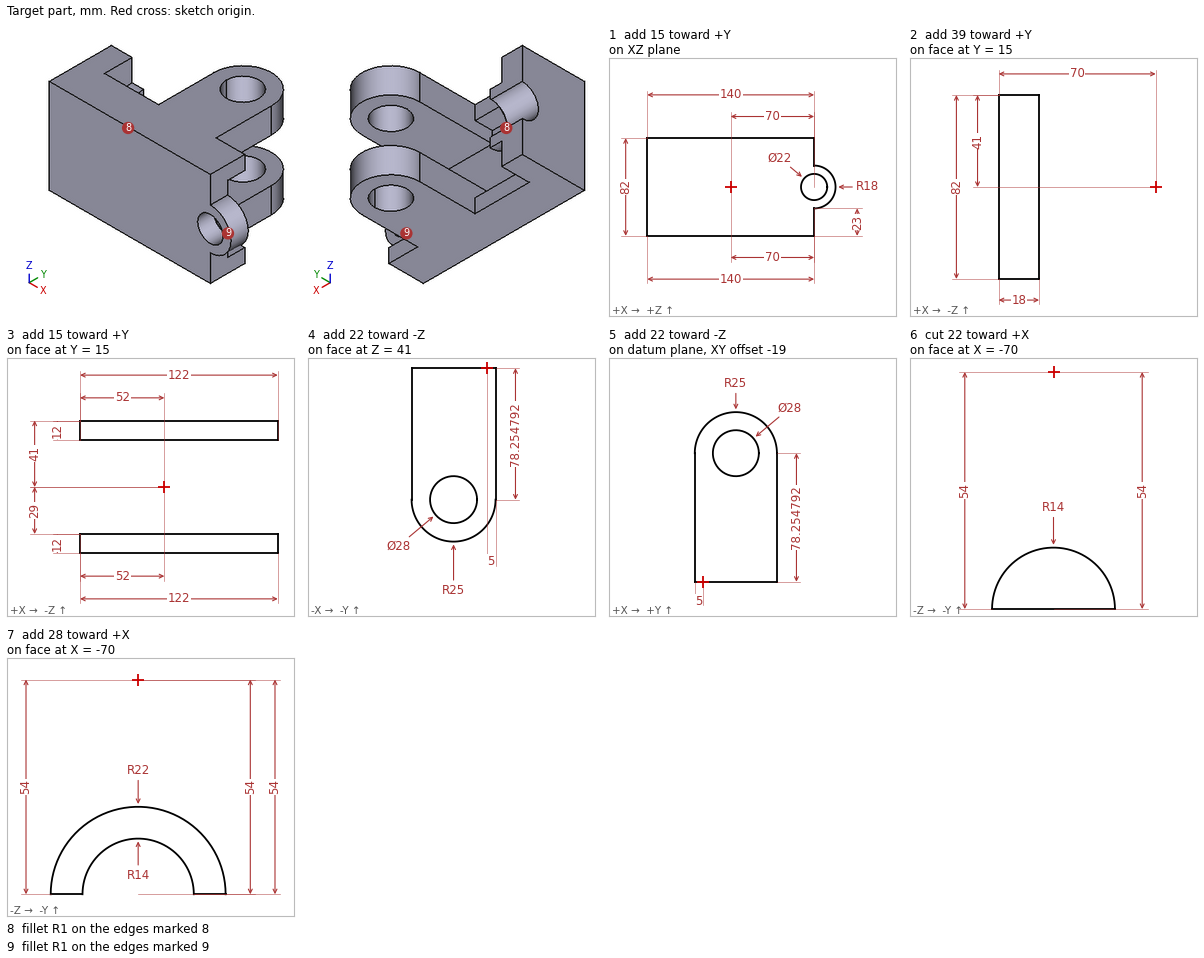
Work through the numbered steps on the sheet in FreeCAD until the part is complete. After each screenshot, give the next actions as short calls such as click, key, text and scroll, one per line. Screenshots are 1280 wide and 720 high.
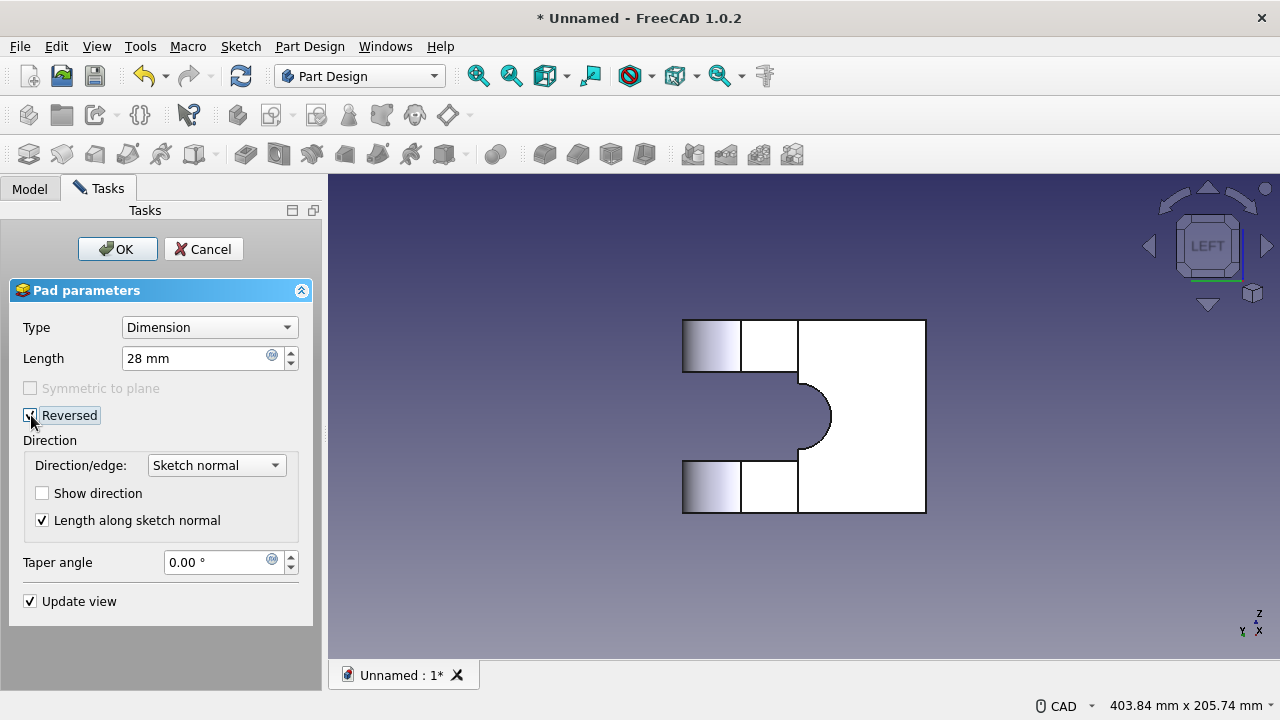
click(118, 249)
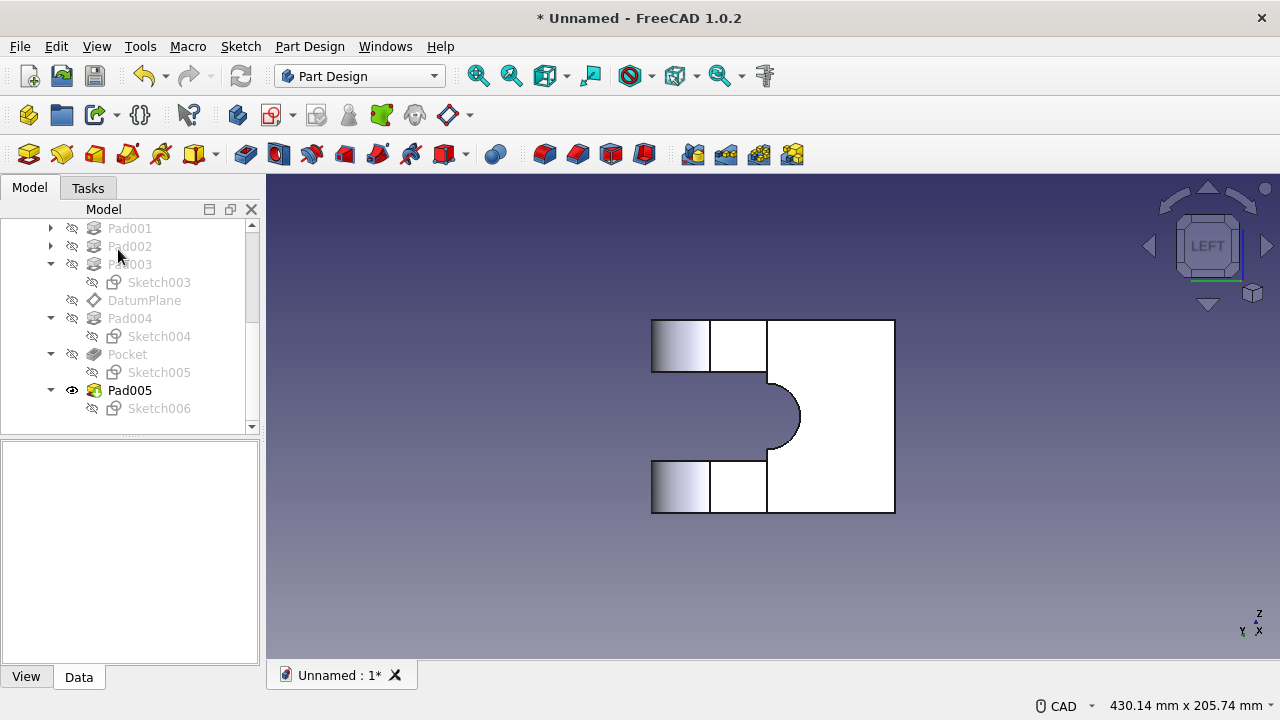
click(479, 76)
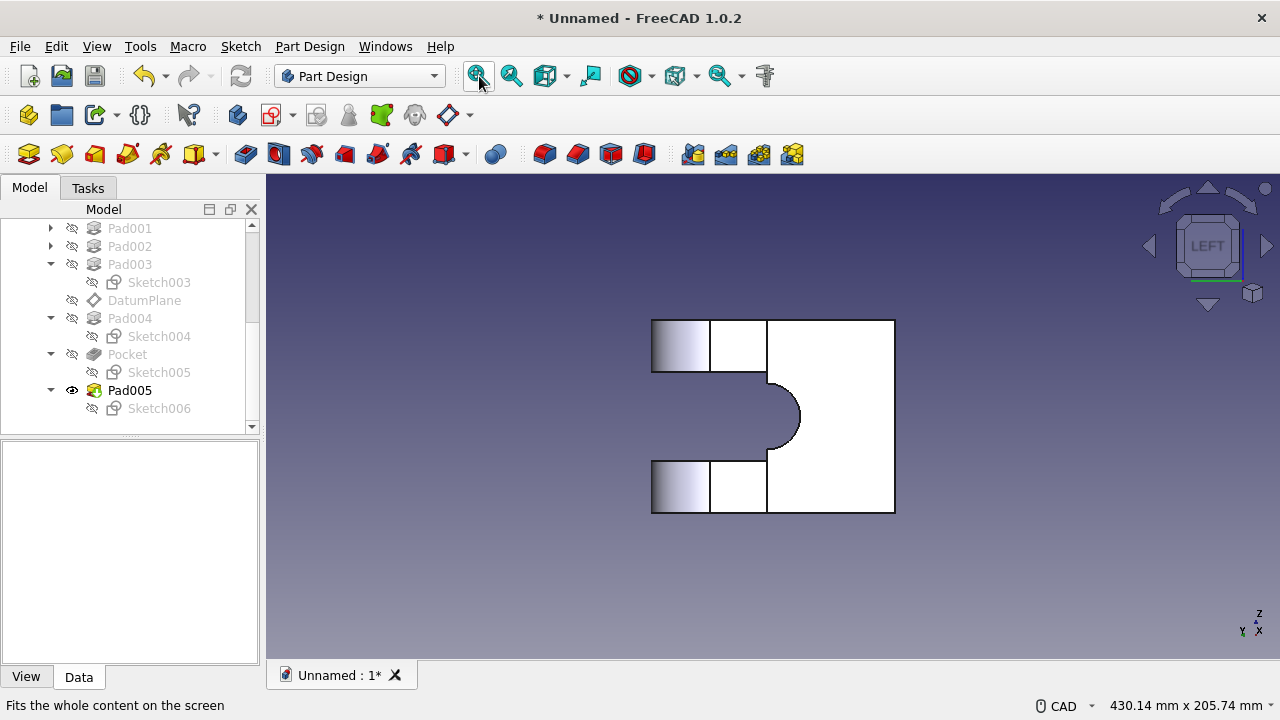
key(0)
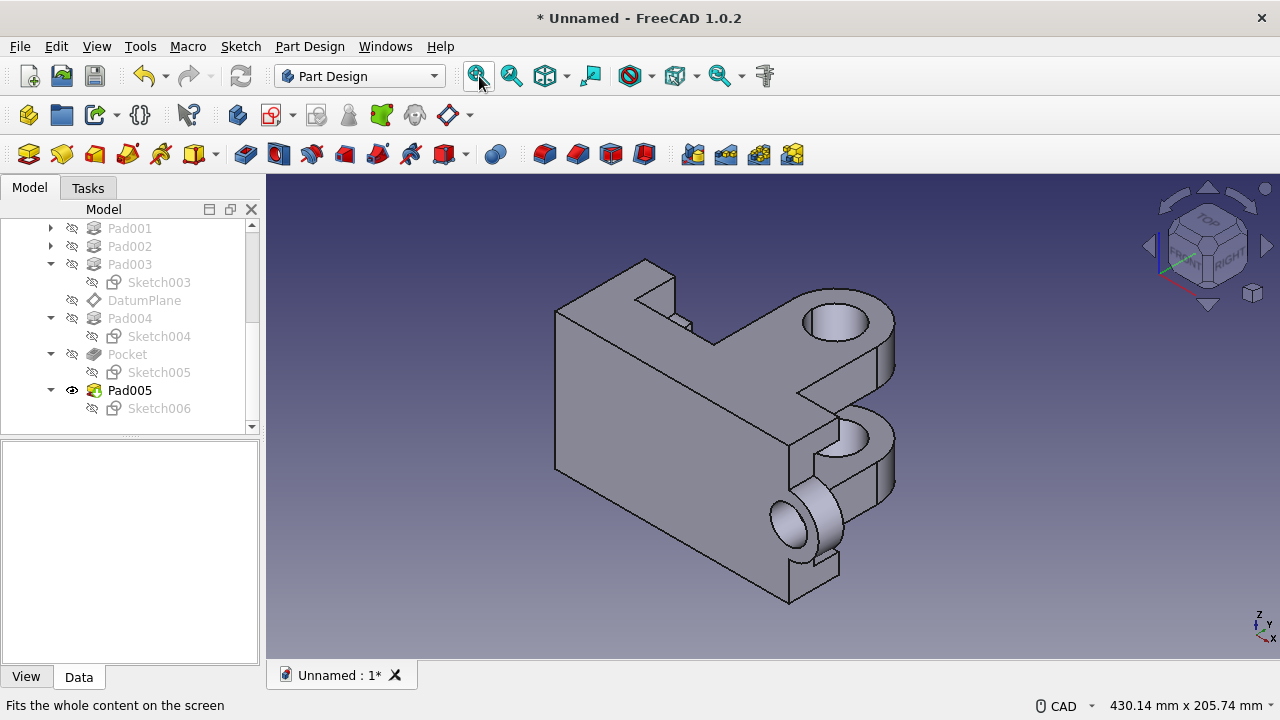
key(2)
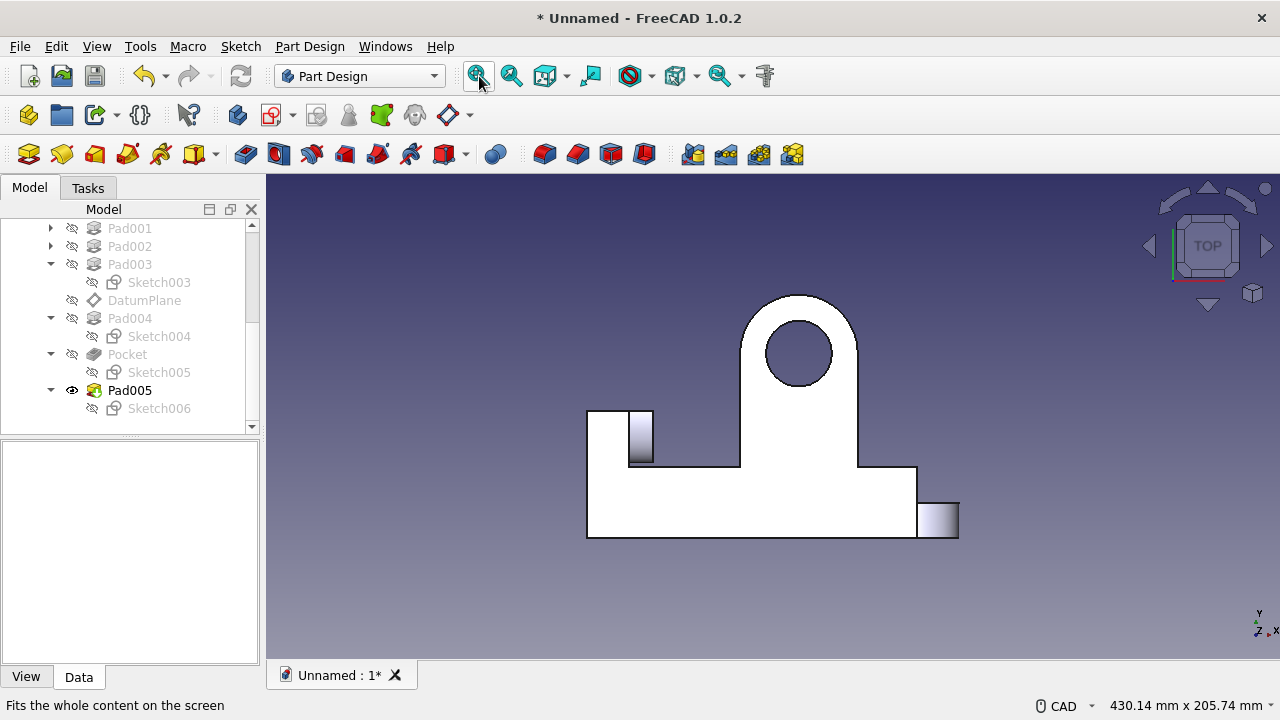
key(1)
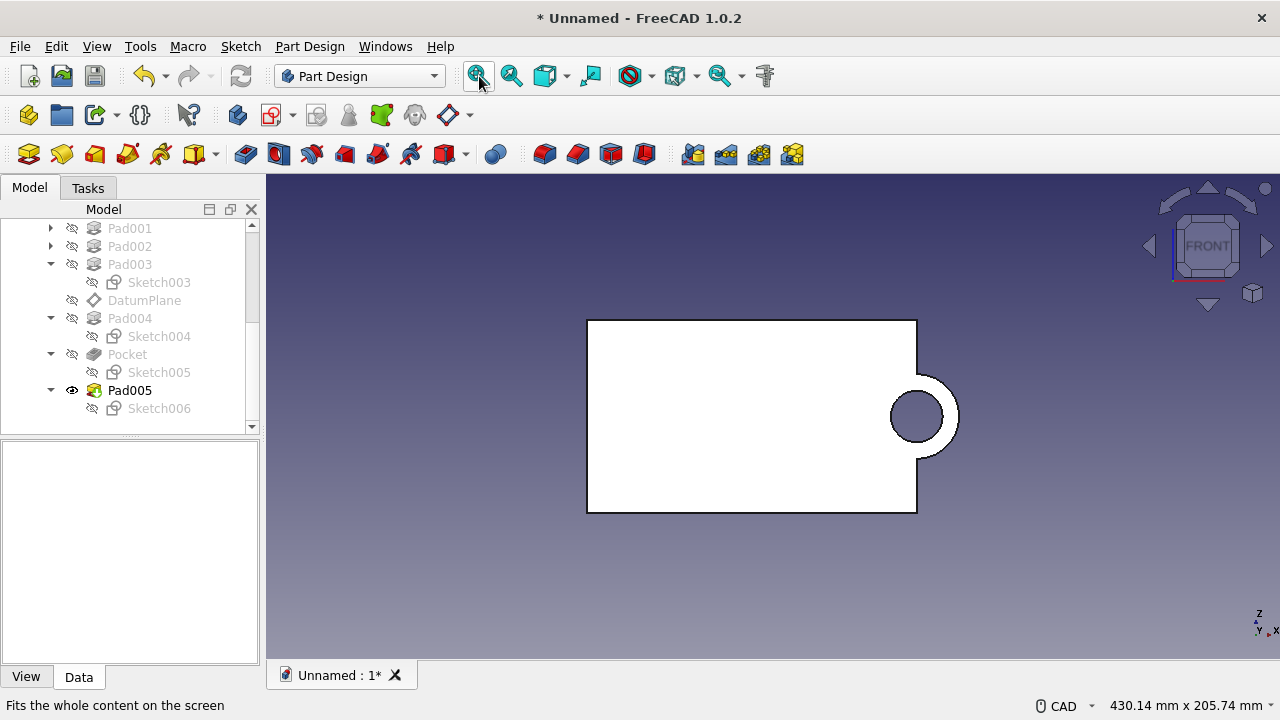
click(479, 76)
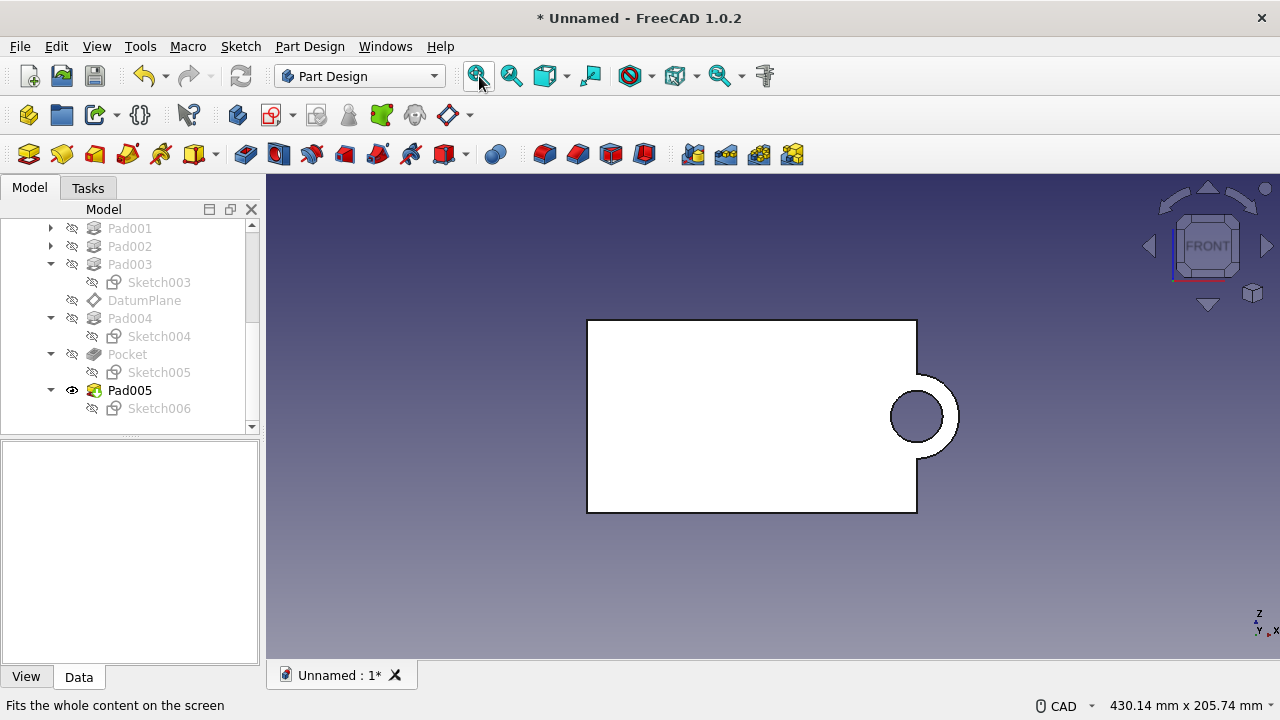
key(3)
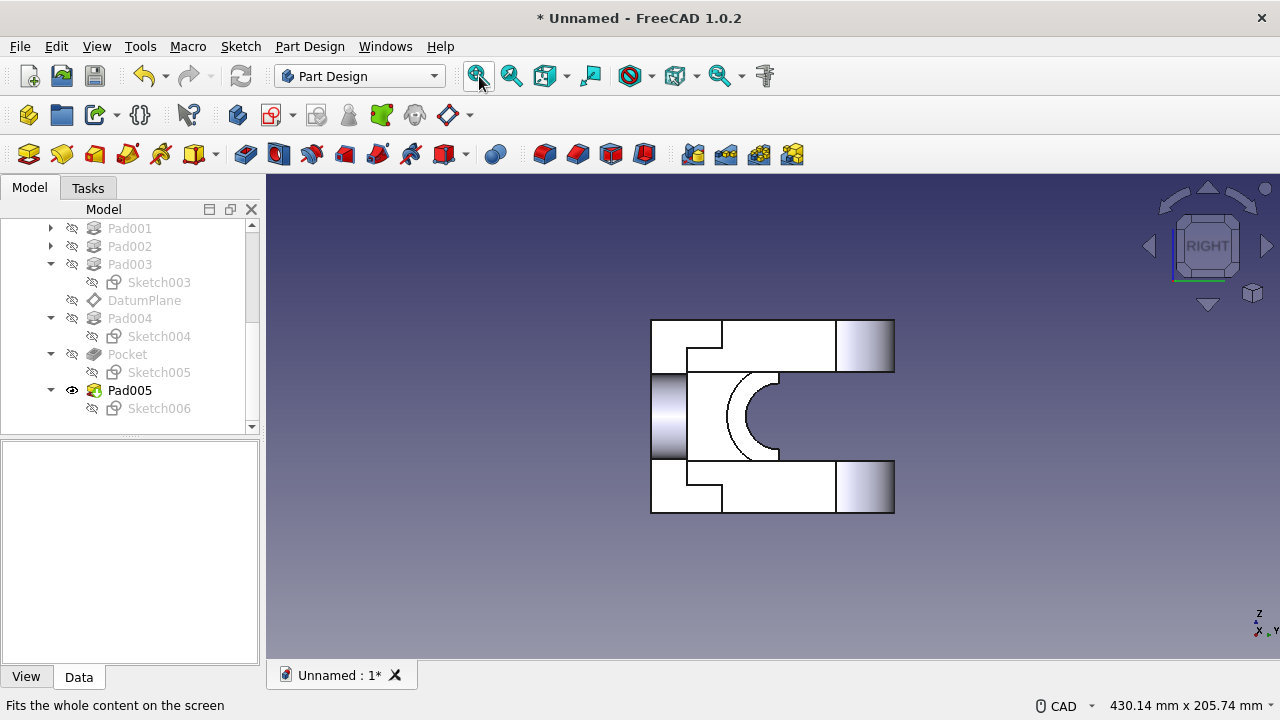
click(479, 76)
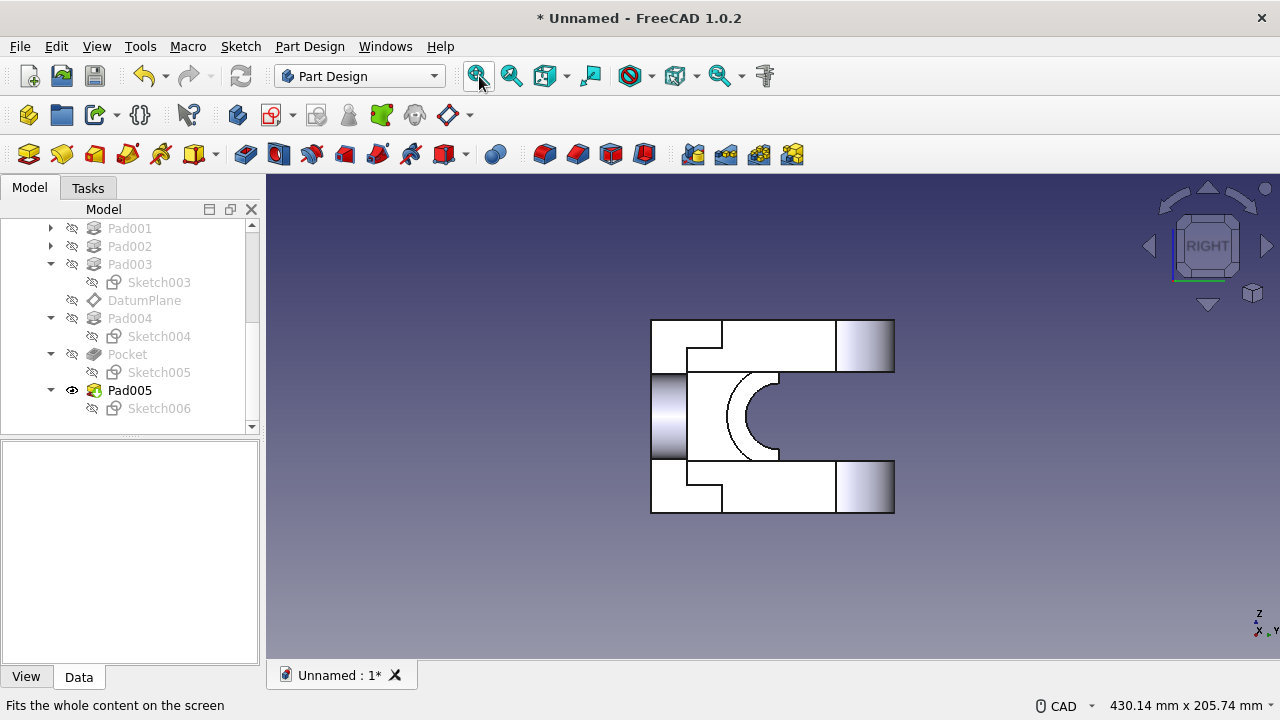
click(746, 416)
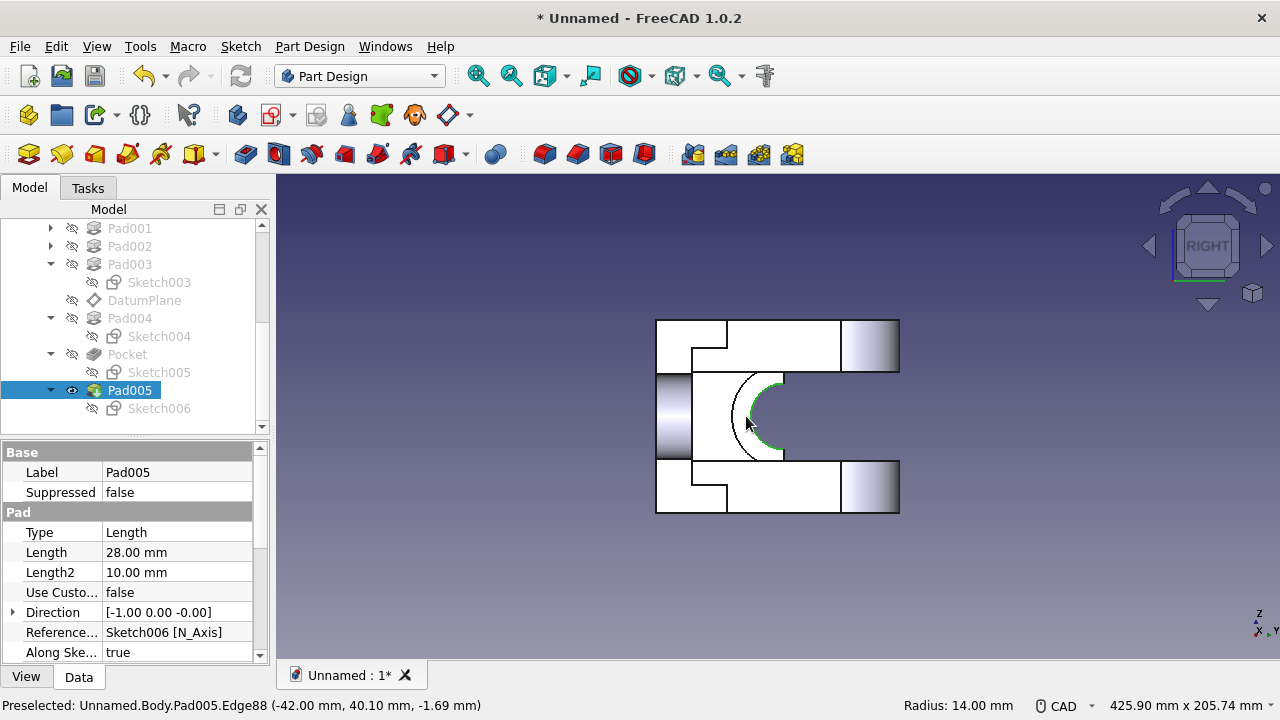
click(545, 154)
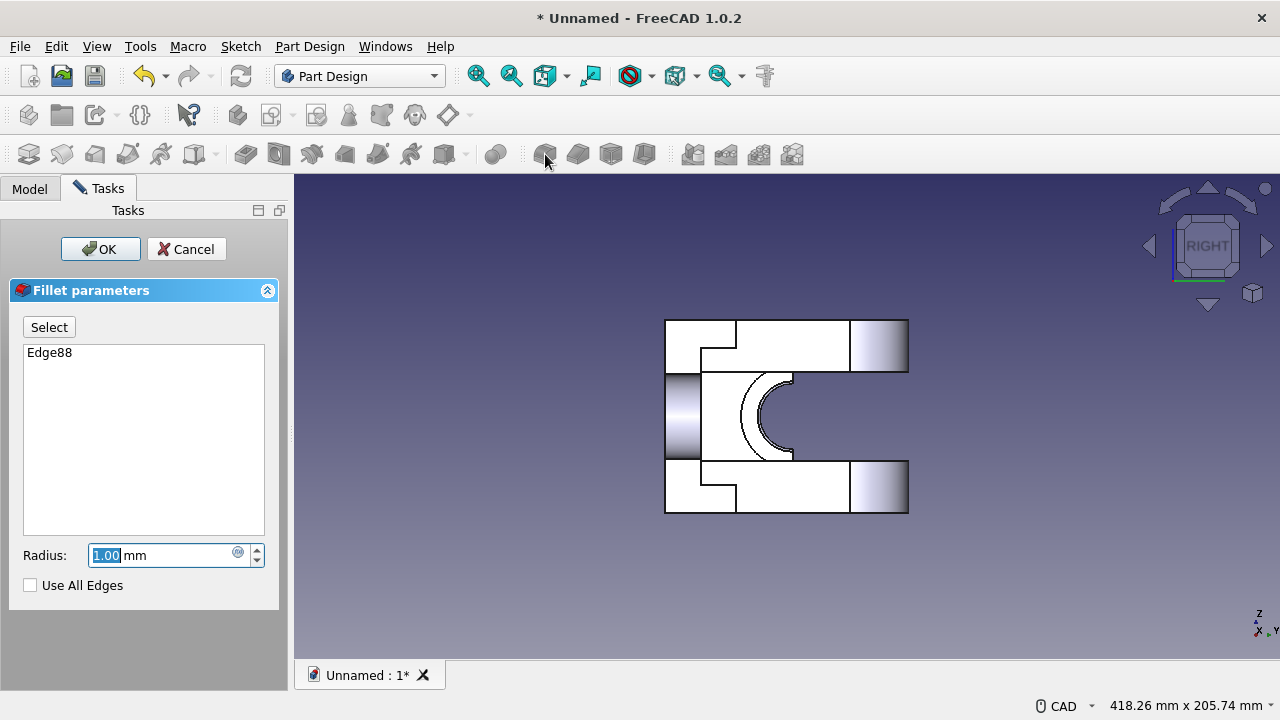
text(1)
key(Tab)